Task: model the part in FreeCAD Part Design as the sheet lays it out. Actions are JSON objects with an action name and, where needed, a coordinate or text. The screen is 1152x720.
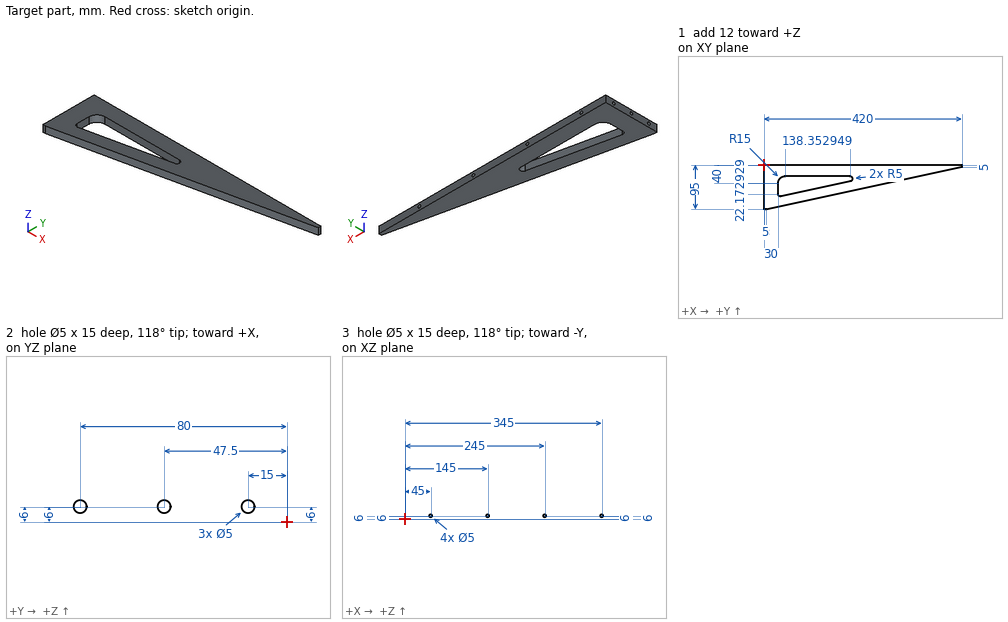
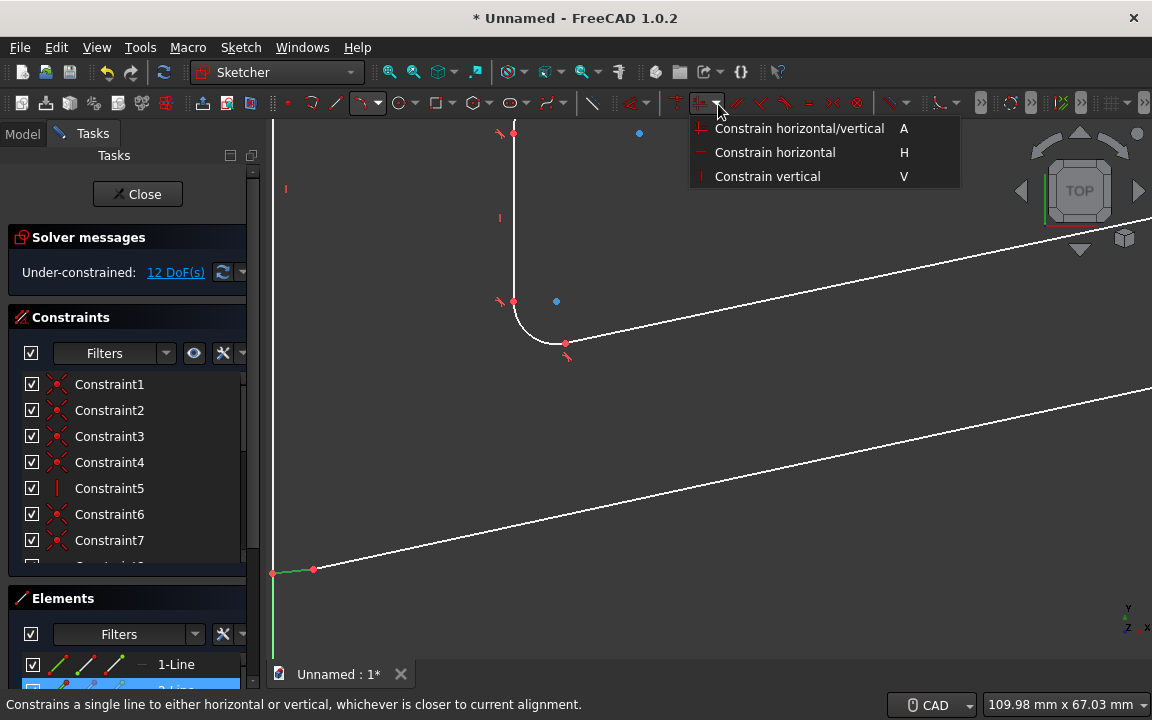
{"action": "left_click", "coordinate": [825, 152]}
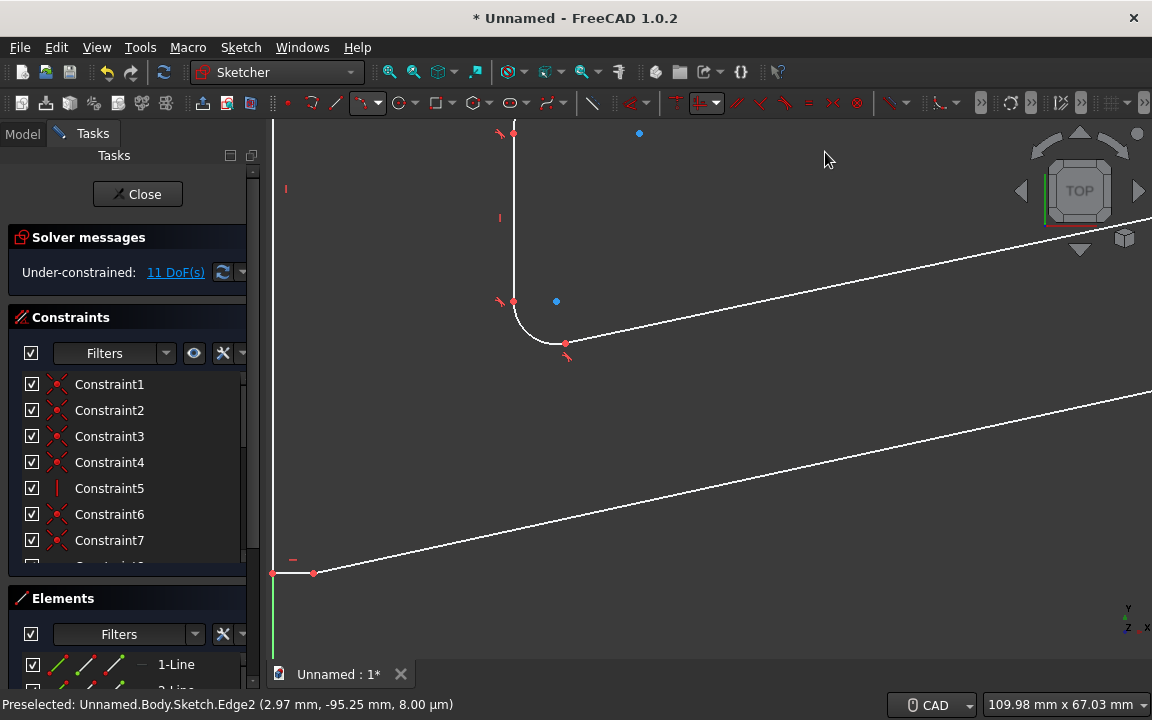
{"action": "scroll", "coordinate": [433, 421], "scroll_direction": "down", "scroll_amount": 10}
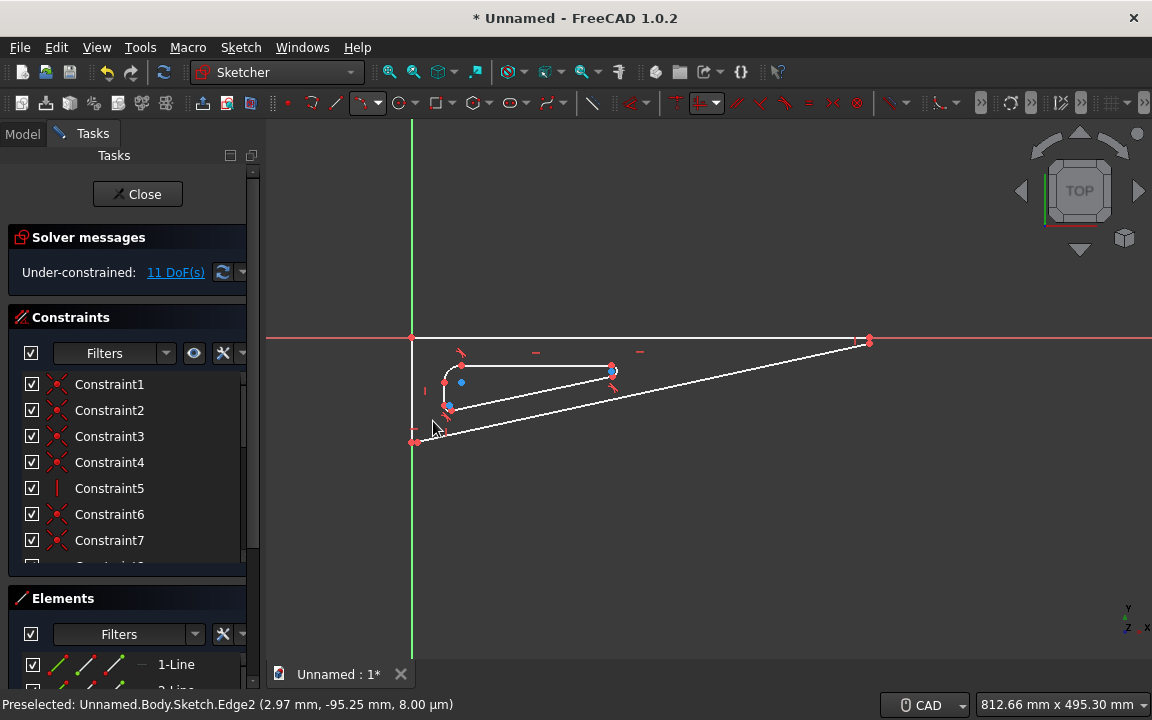
{"action": "scroll", "coordinate": [616, 374], "scroll_direction": "up", "scroll_amount": 6}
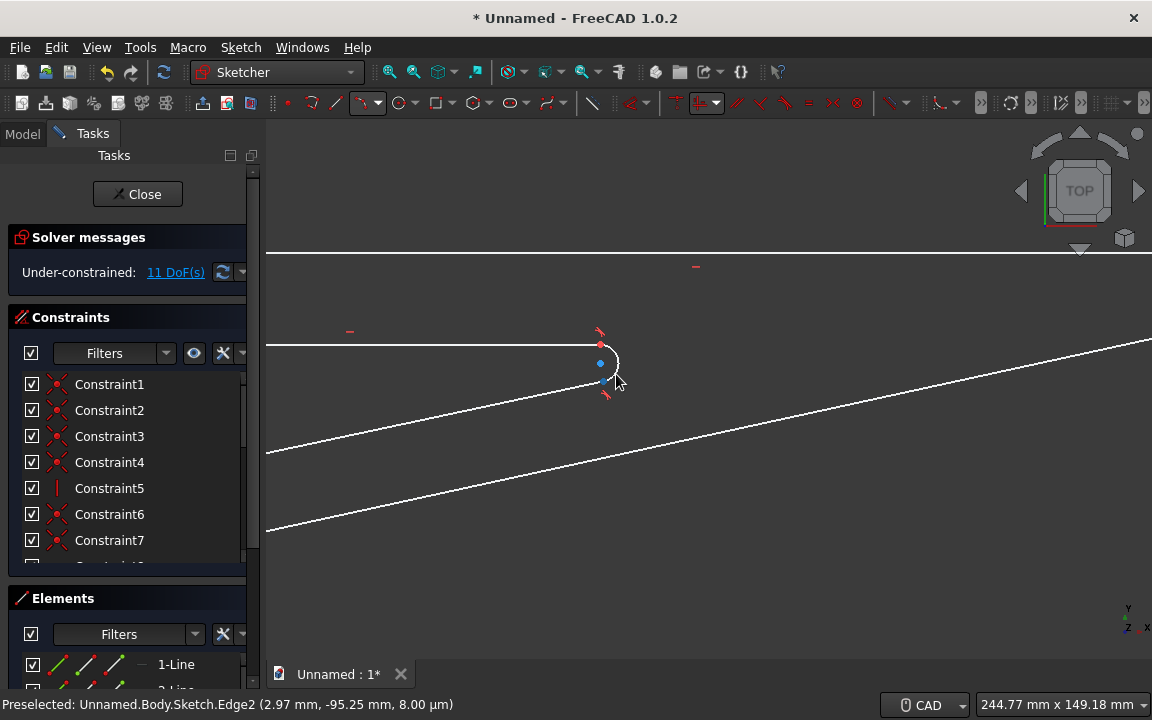
{"action": "left_click", "coordinate": [616, 372]}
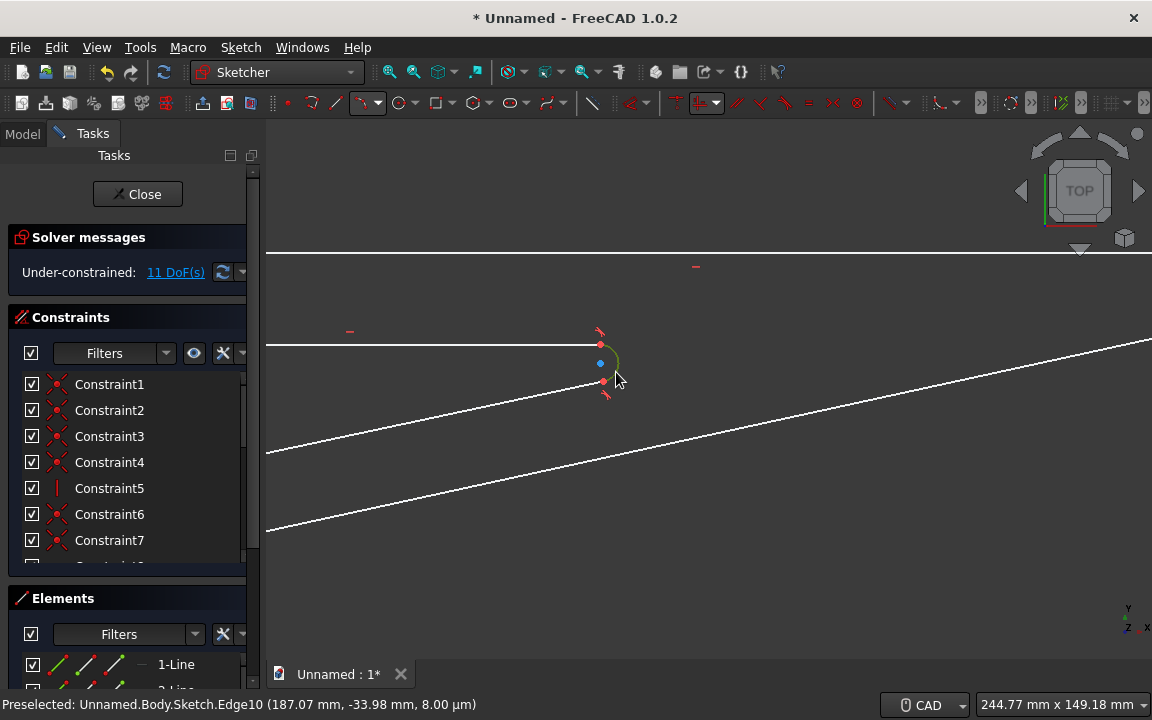
{"action": "scroll", "coordinate": [616, 373], "scroll_direction": "down", "scroll_amount": 6}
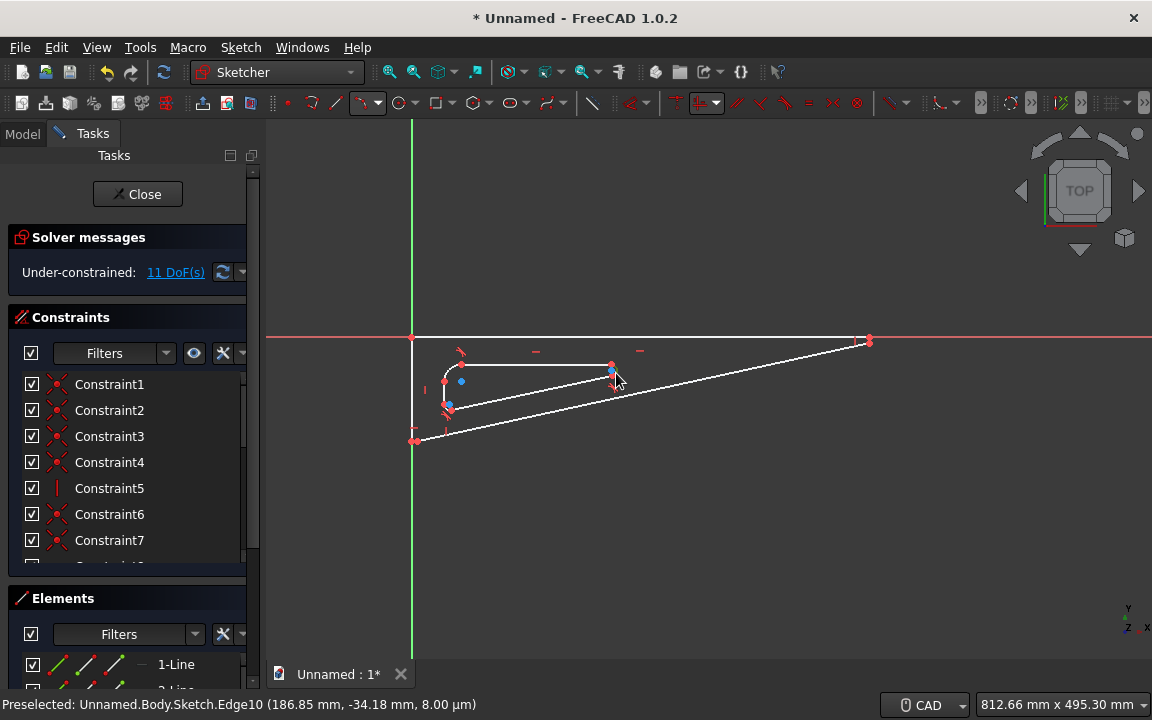
{"action": "scroll", "coordinate": [445, 408], "scroll_direction": "up", "scroll_amount": 8}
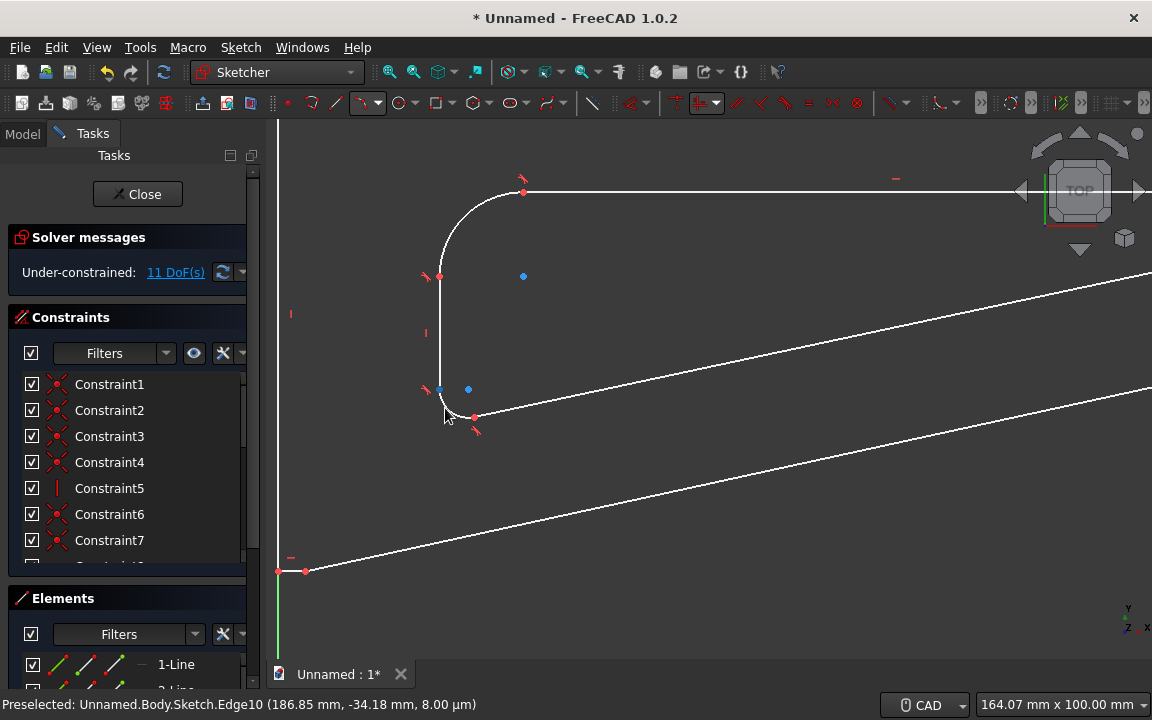
{"action": "left_click", "coordinate": [444, 404]}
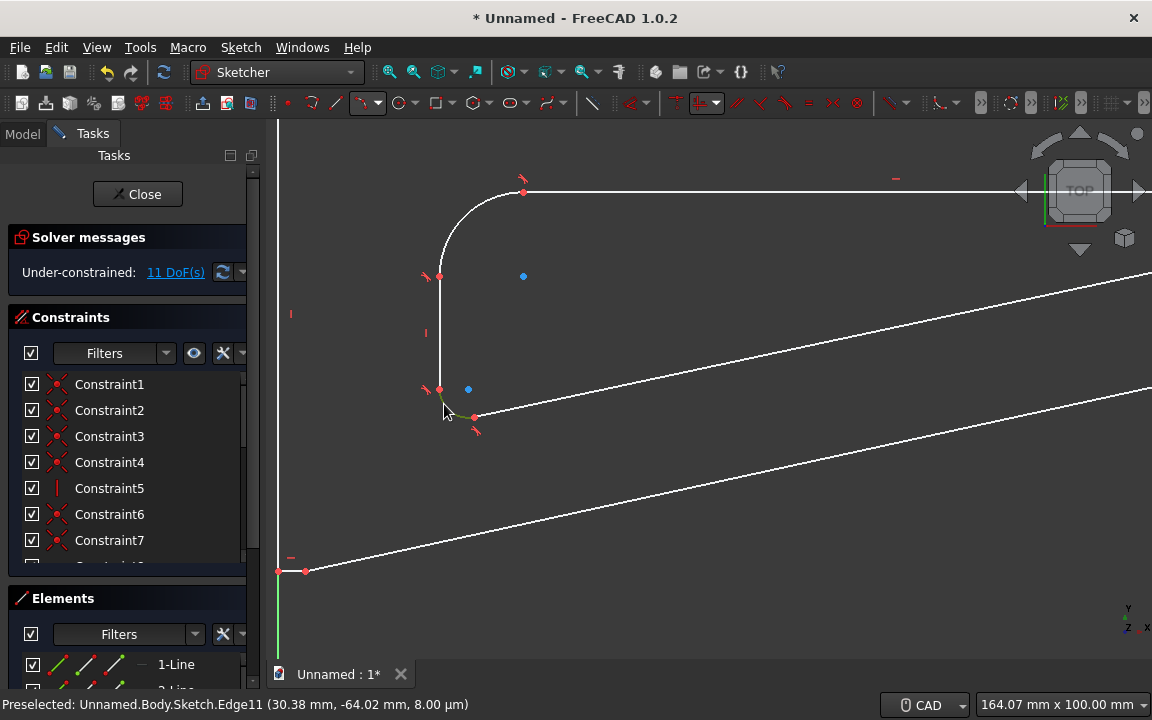
{"action": "left_click", "coordinate": [810, 104]}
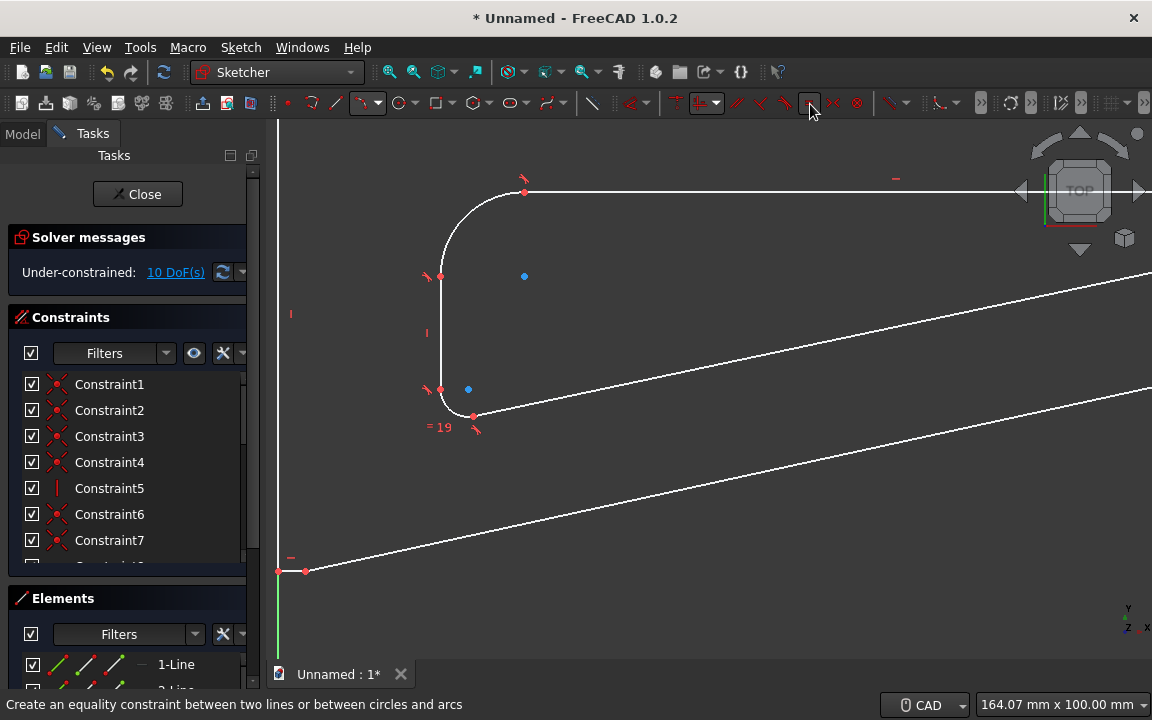
{"action": "left_click", "coordinate": [486, 201]}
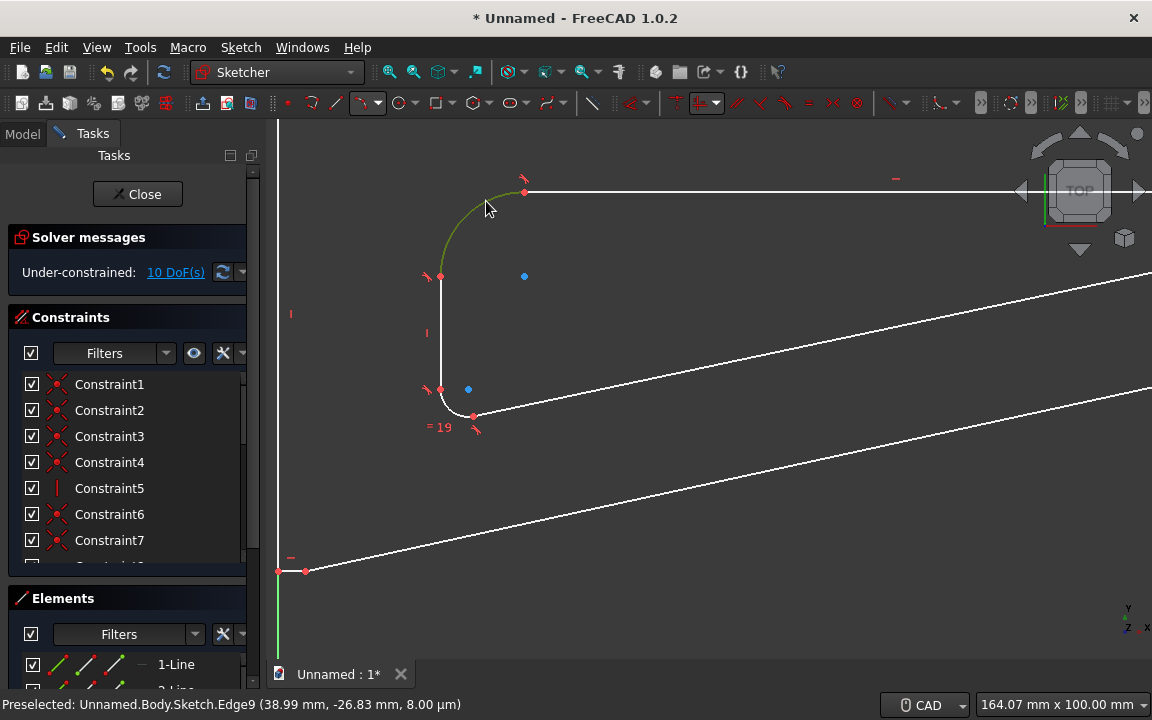
{"action": "left_click", "coordinate": [648, 104]}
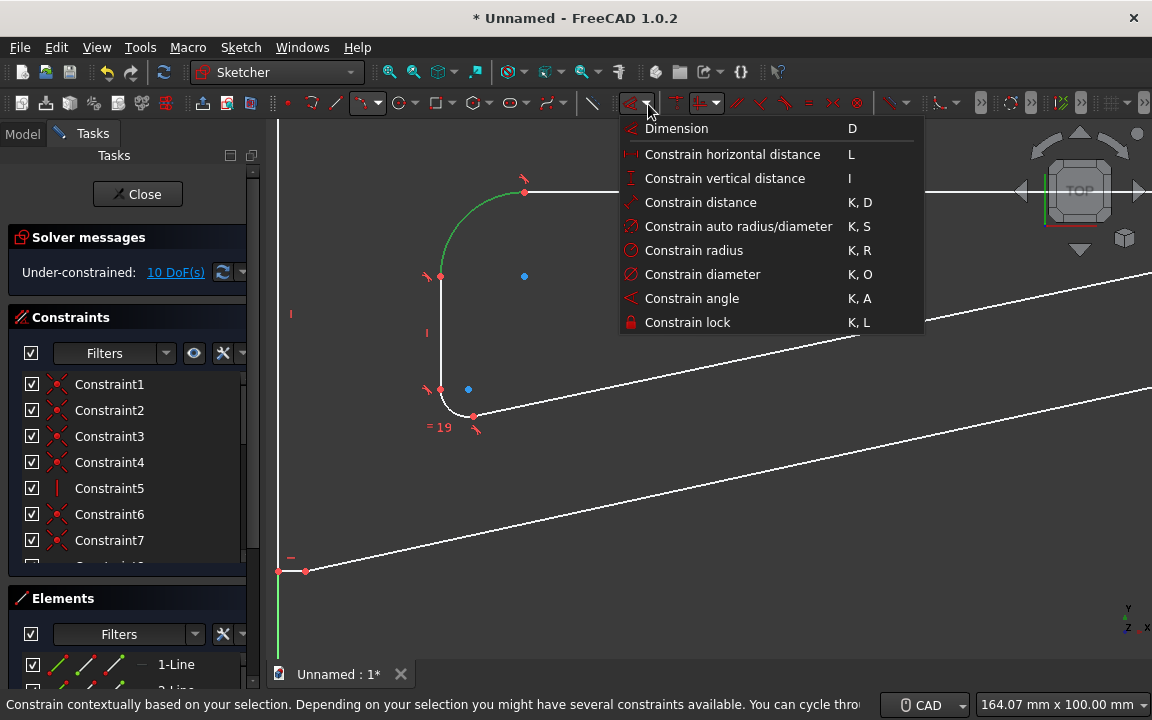
{"action": "left_click", "coordinate": [772, 250]}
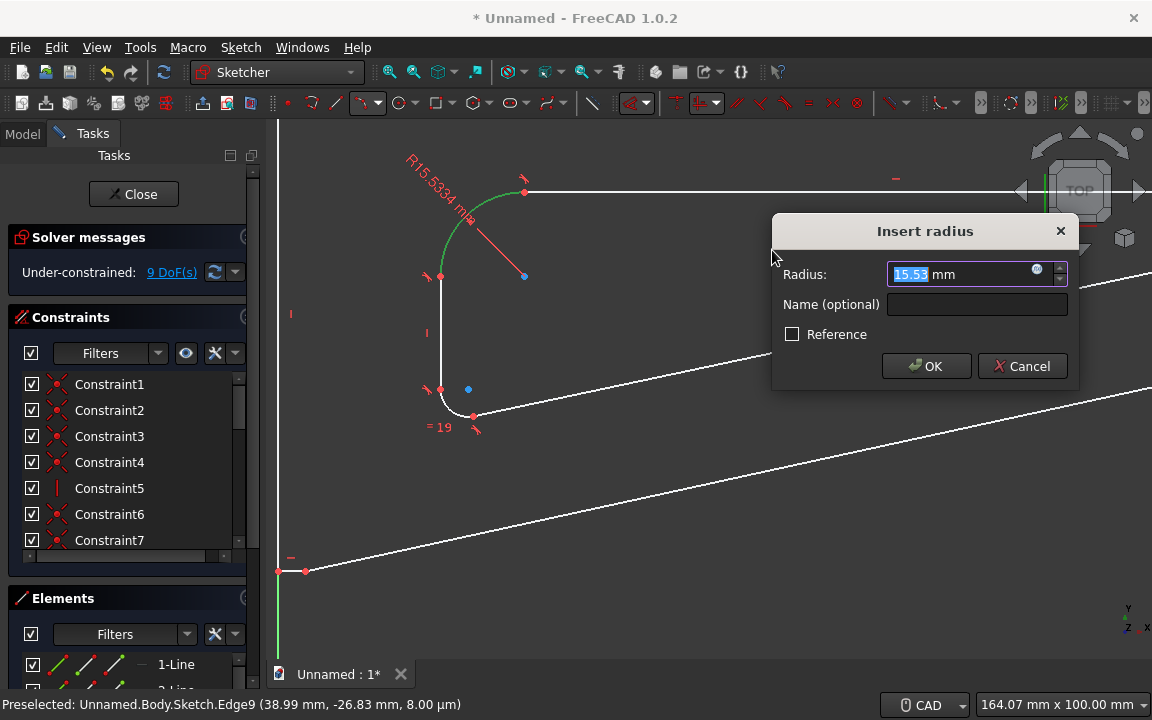
{"action": "type", "text": "15"}
{"action": "key", "text": "Return"}